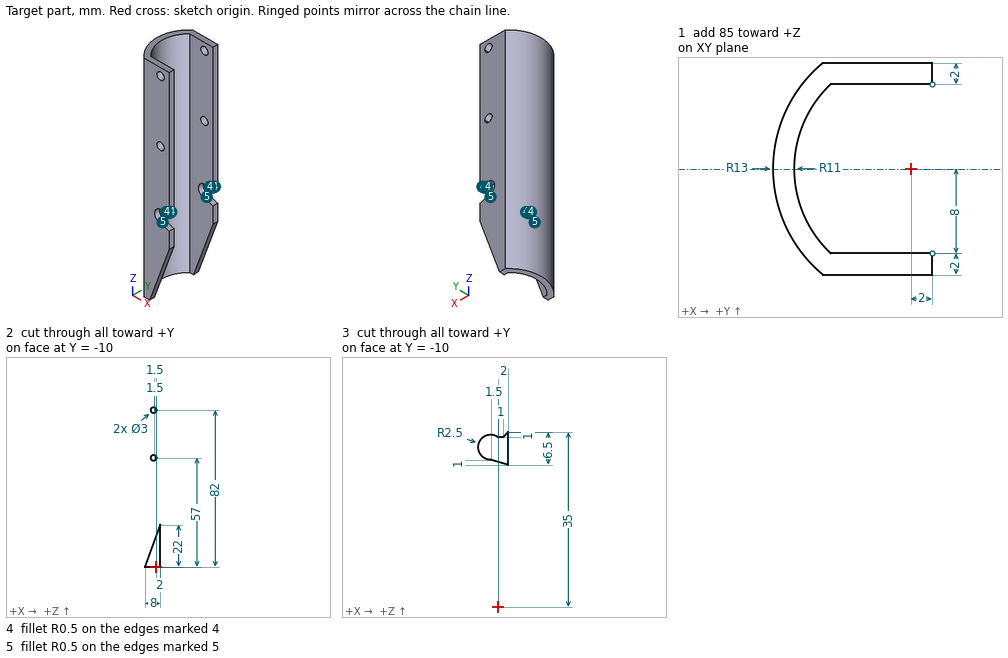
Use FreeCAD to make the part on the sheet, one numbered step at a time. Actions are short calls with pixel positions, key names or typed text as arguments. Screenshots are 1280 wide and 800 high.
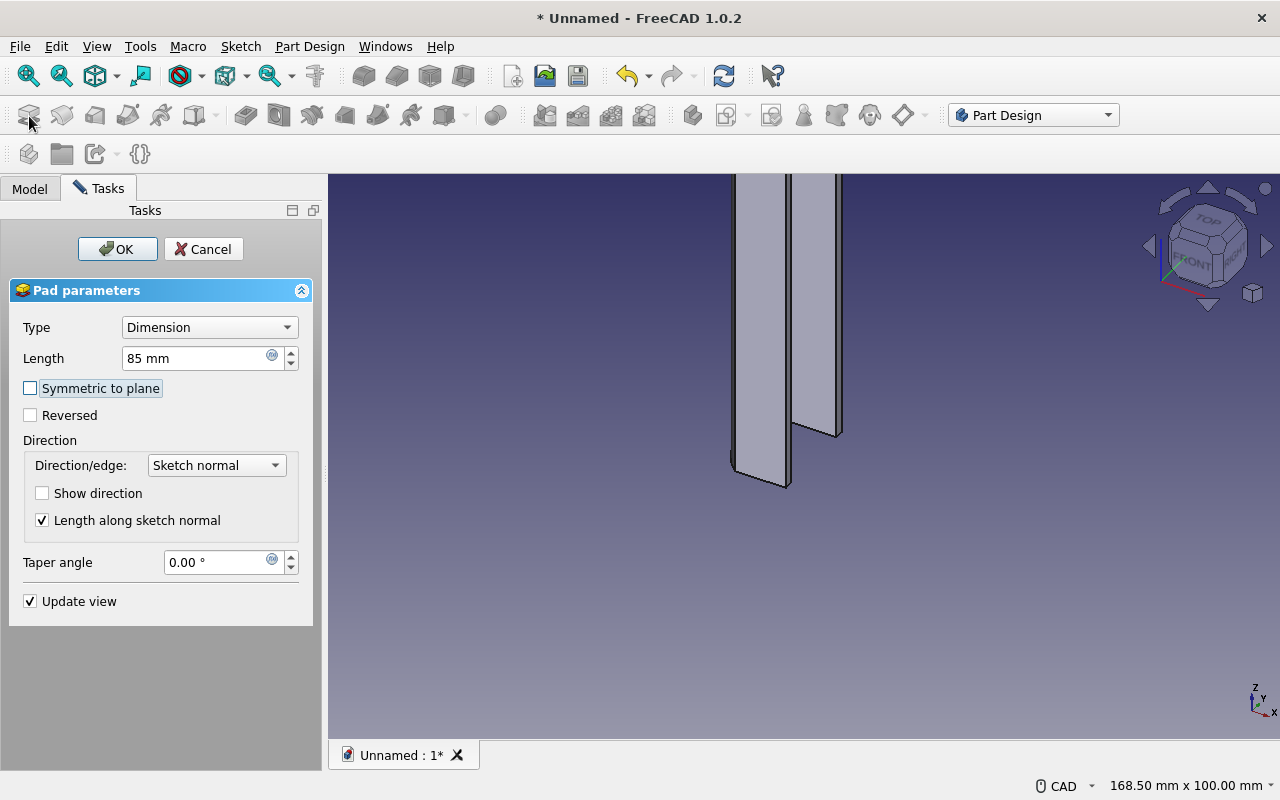
click(118, 249)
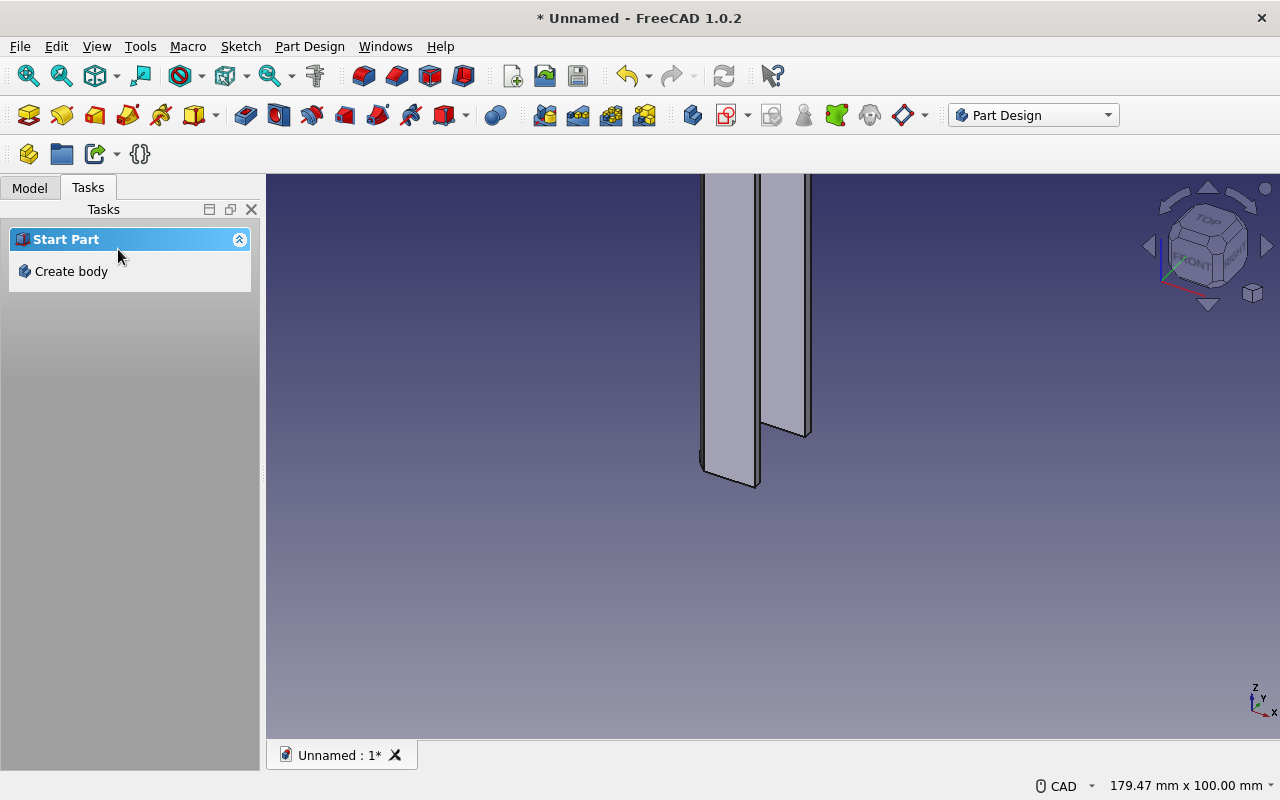
click(29, 76)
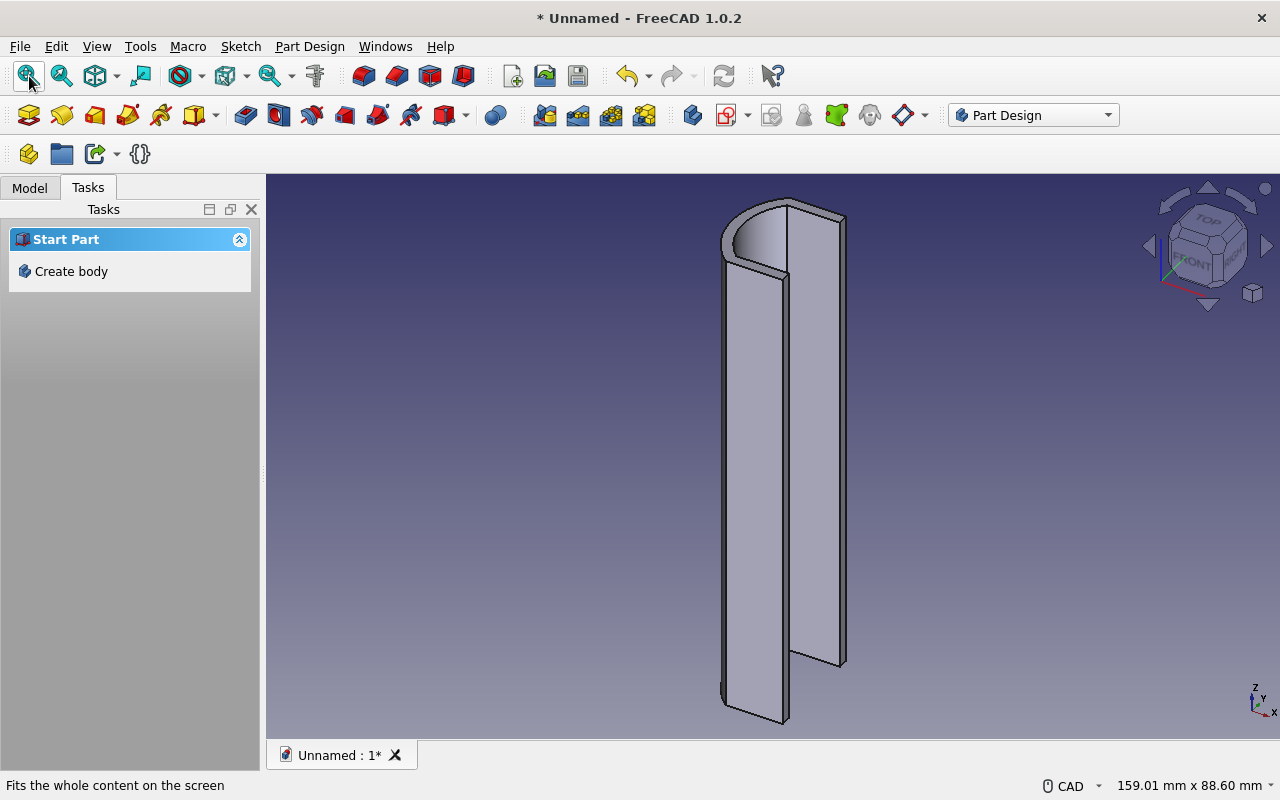
click(754, 301)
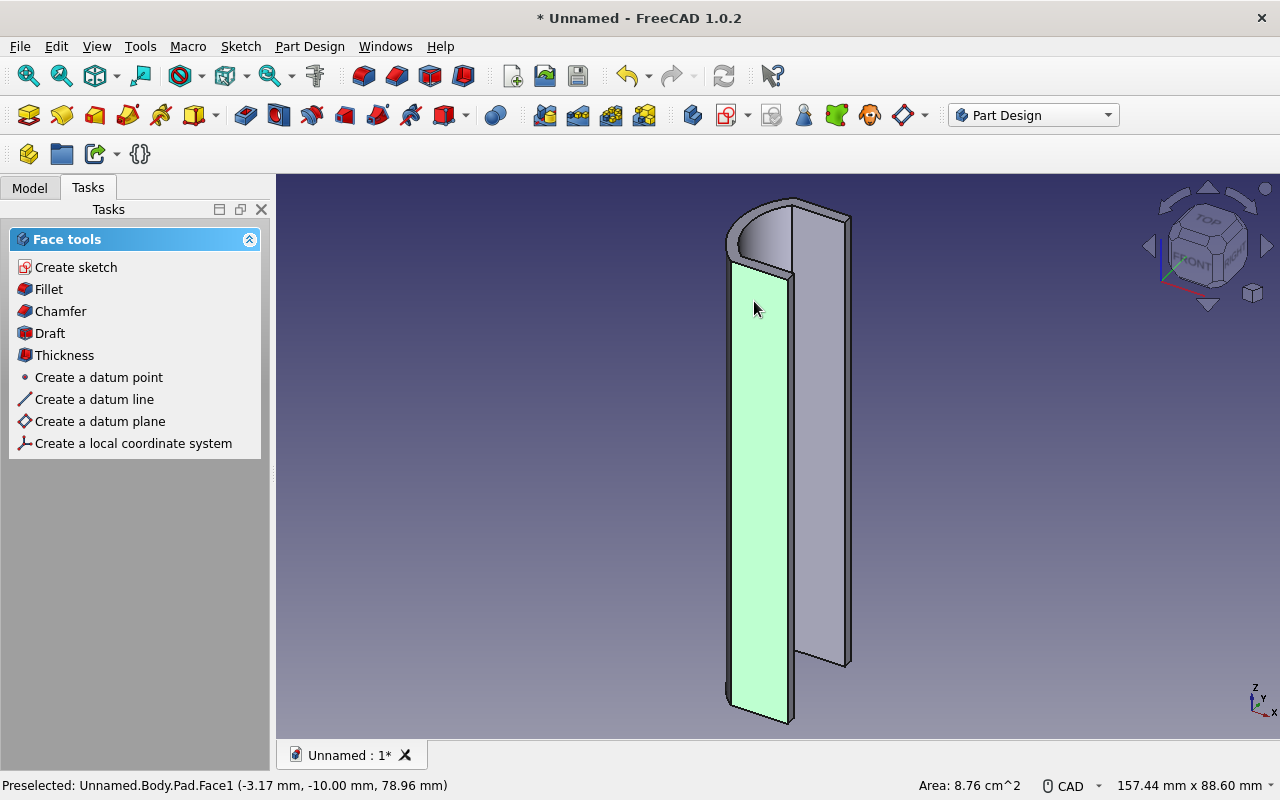
click(726, 116)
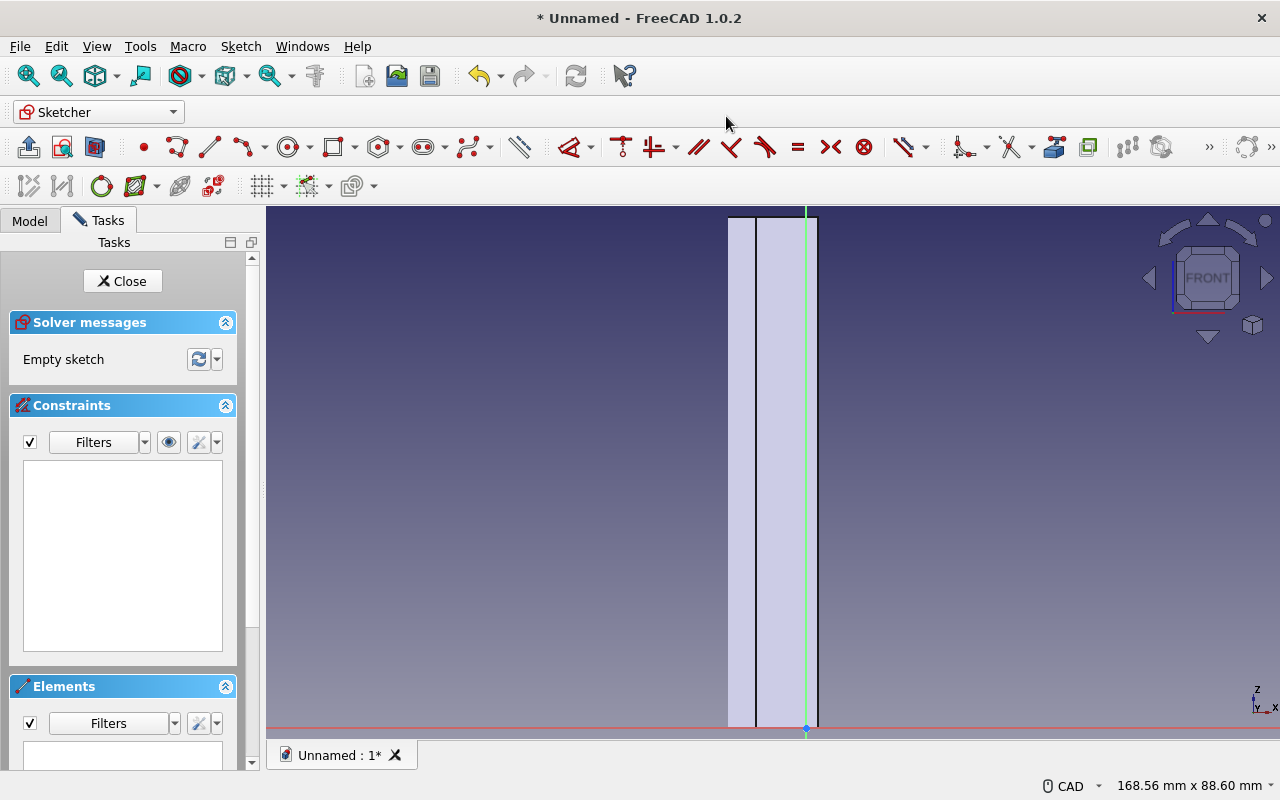
scroll(522, 463, down, 2)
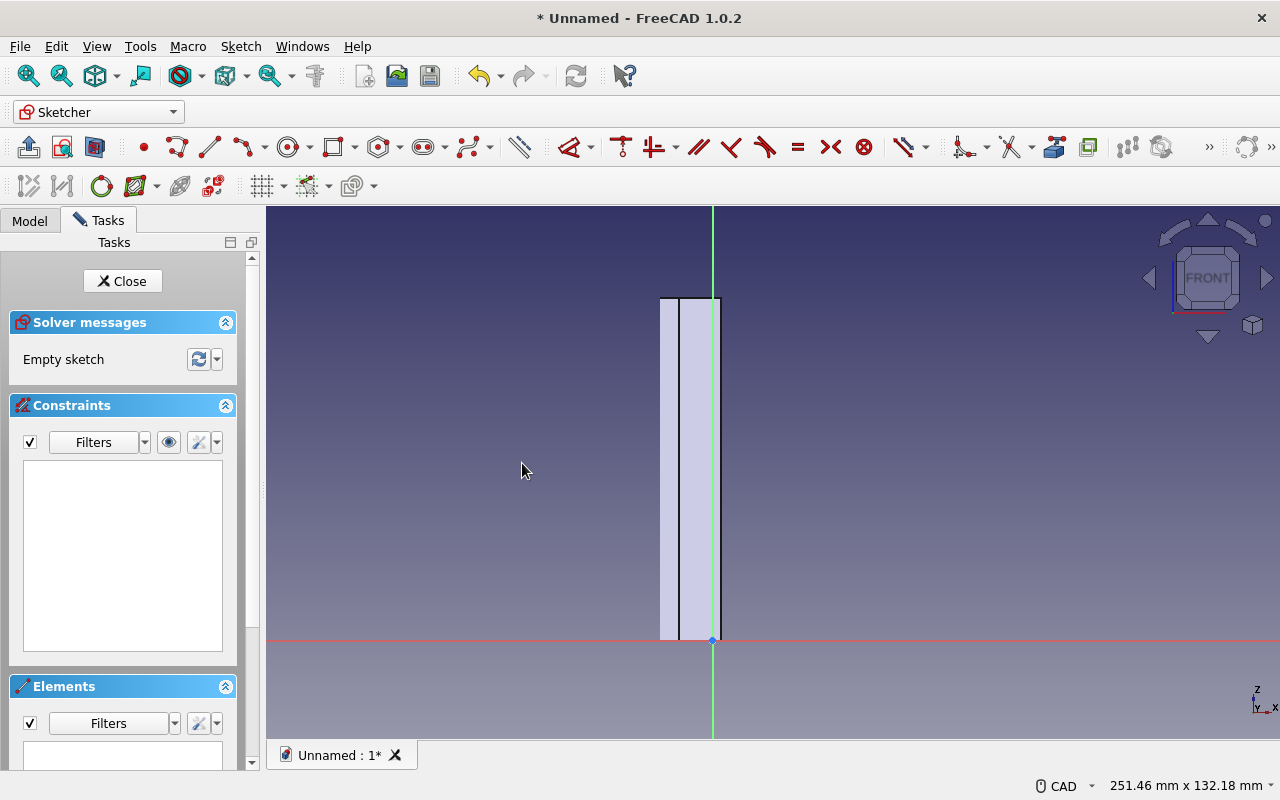
click(177, 148)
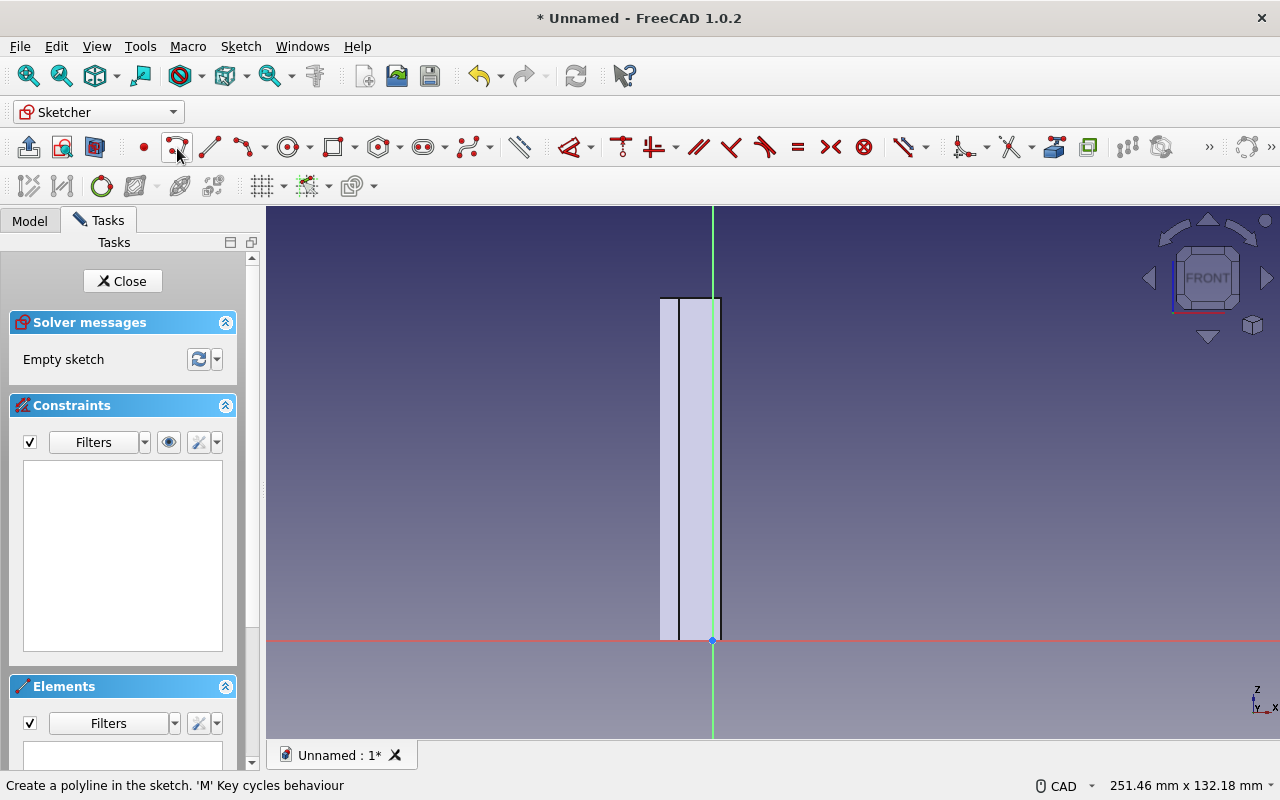
scroll(721, 641, up, 4)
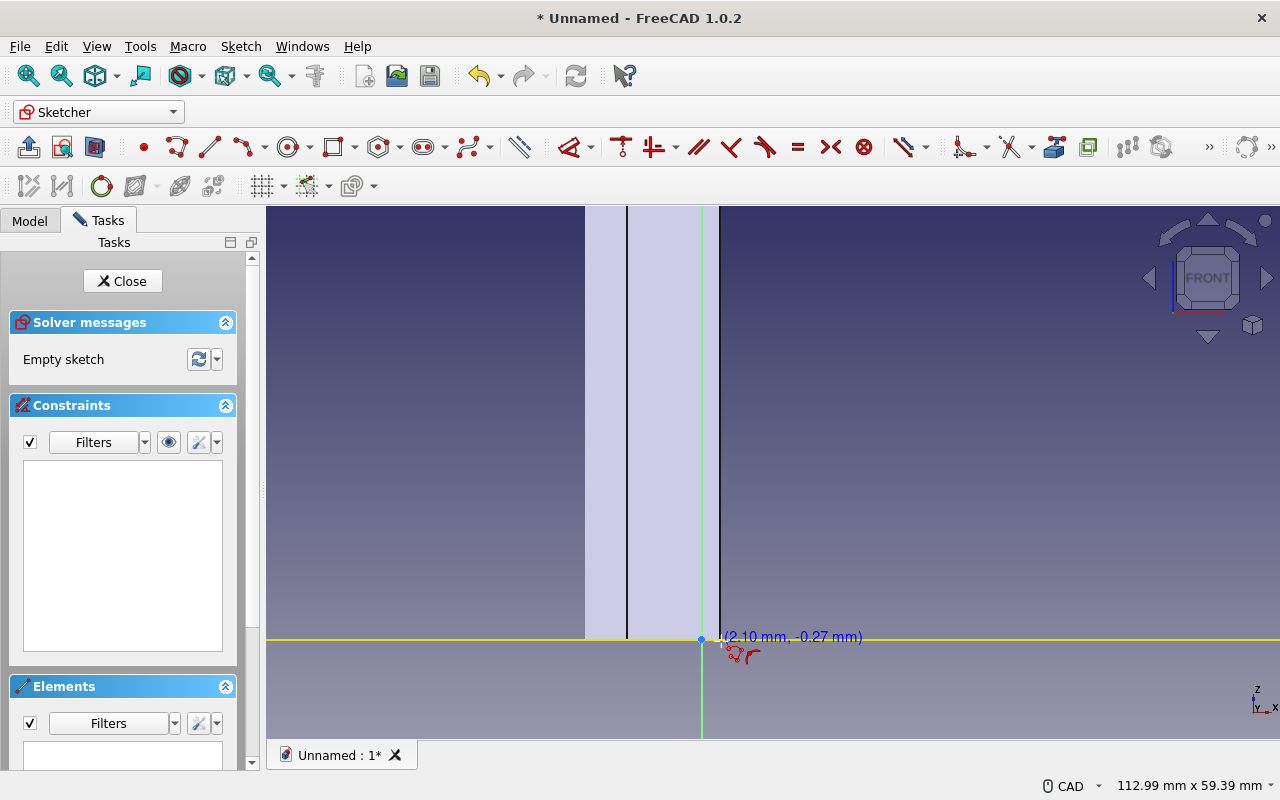
click(720, 640)
click(720, 442)
click(648, 631)
click(720, 640)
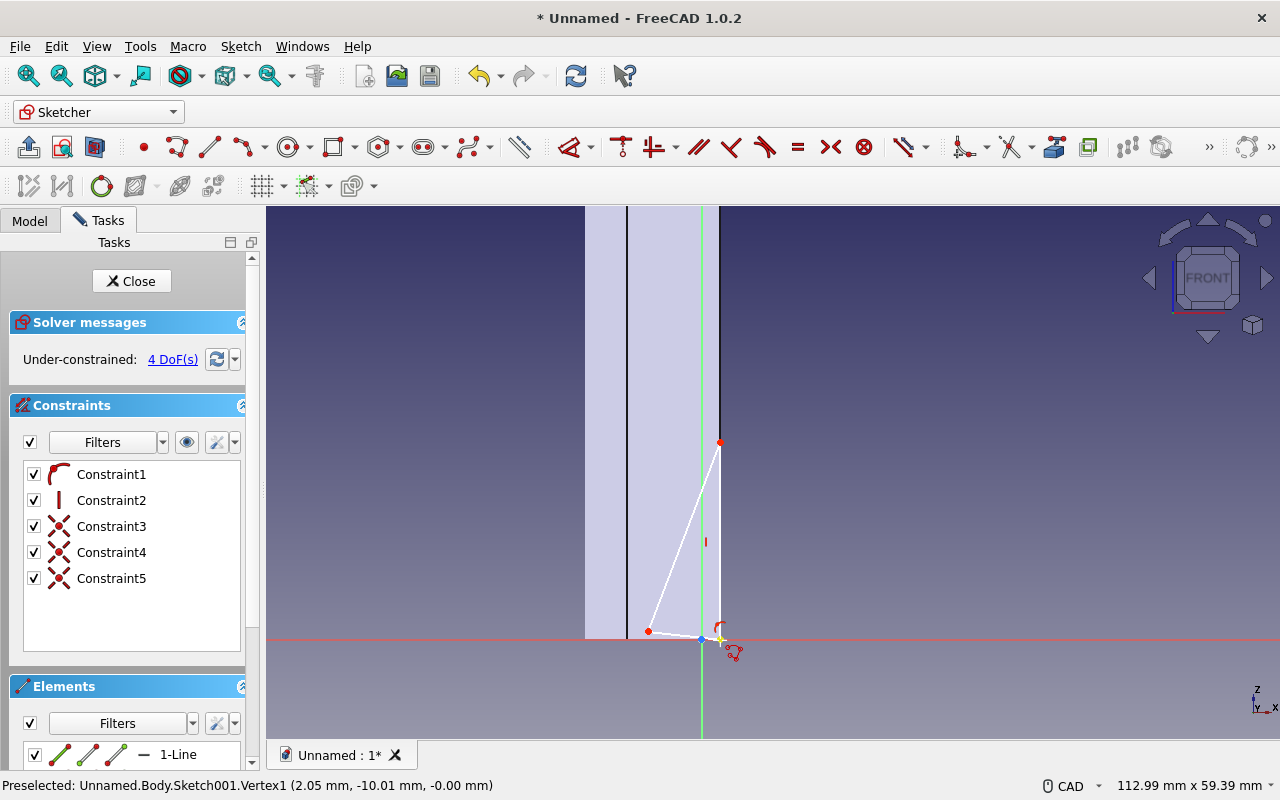
click(288, 148)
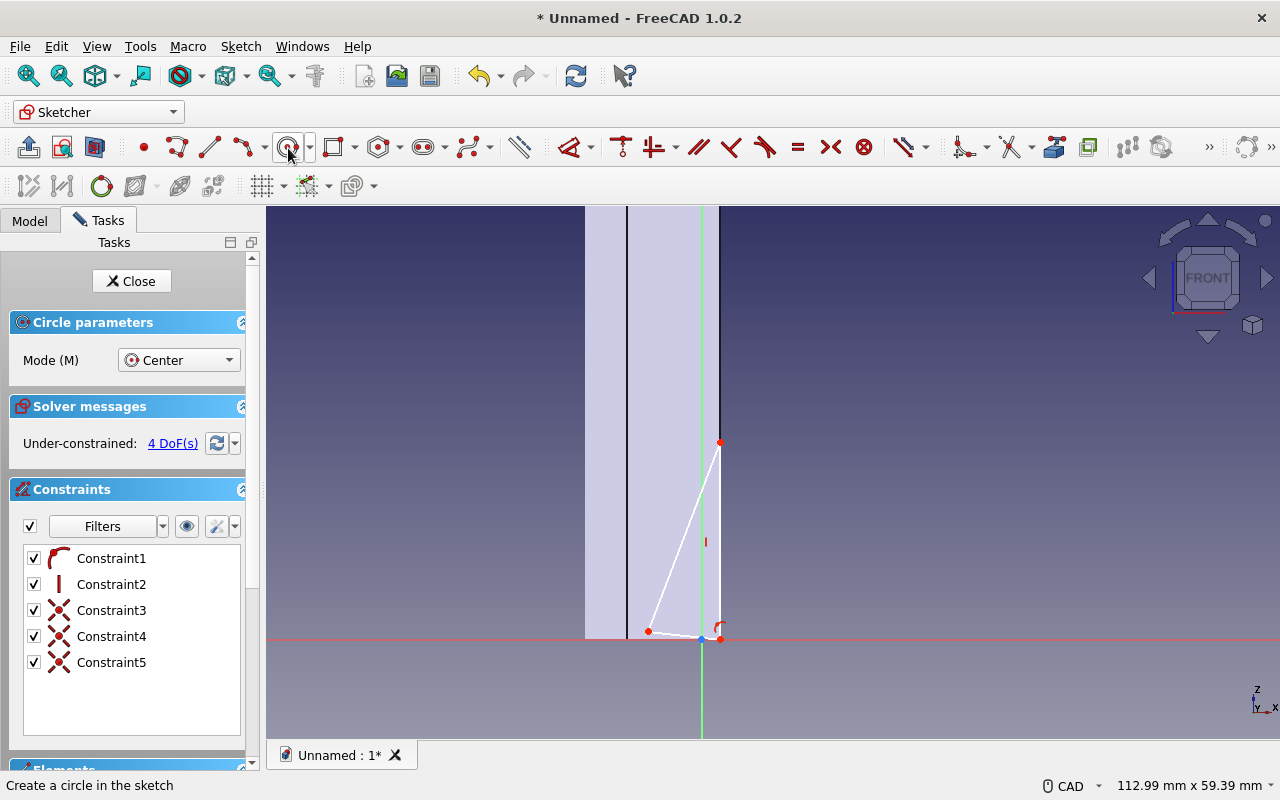
scroll(722, 642, down, 4)